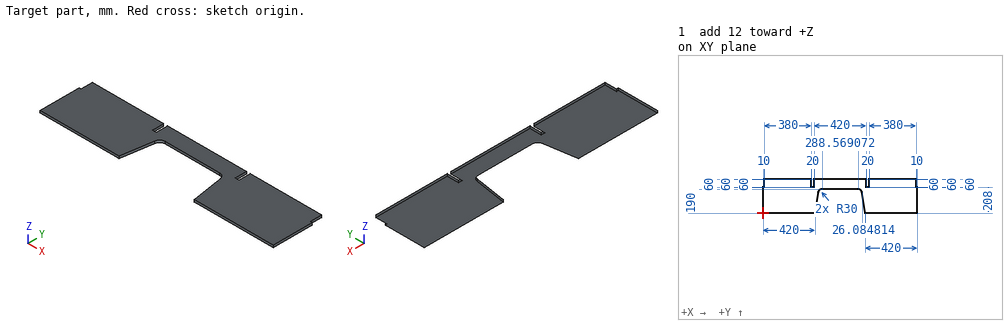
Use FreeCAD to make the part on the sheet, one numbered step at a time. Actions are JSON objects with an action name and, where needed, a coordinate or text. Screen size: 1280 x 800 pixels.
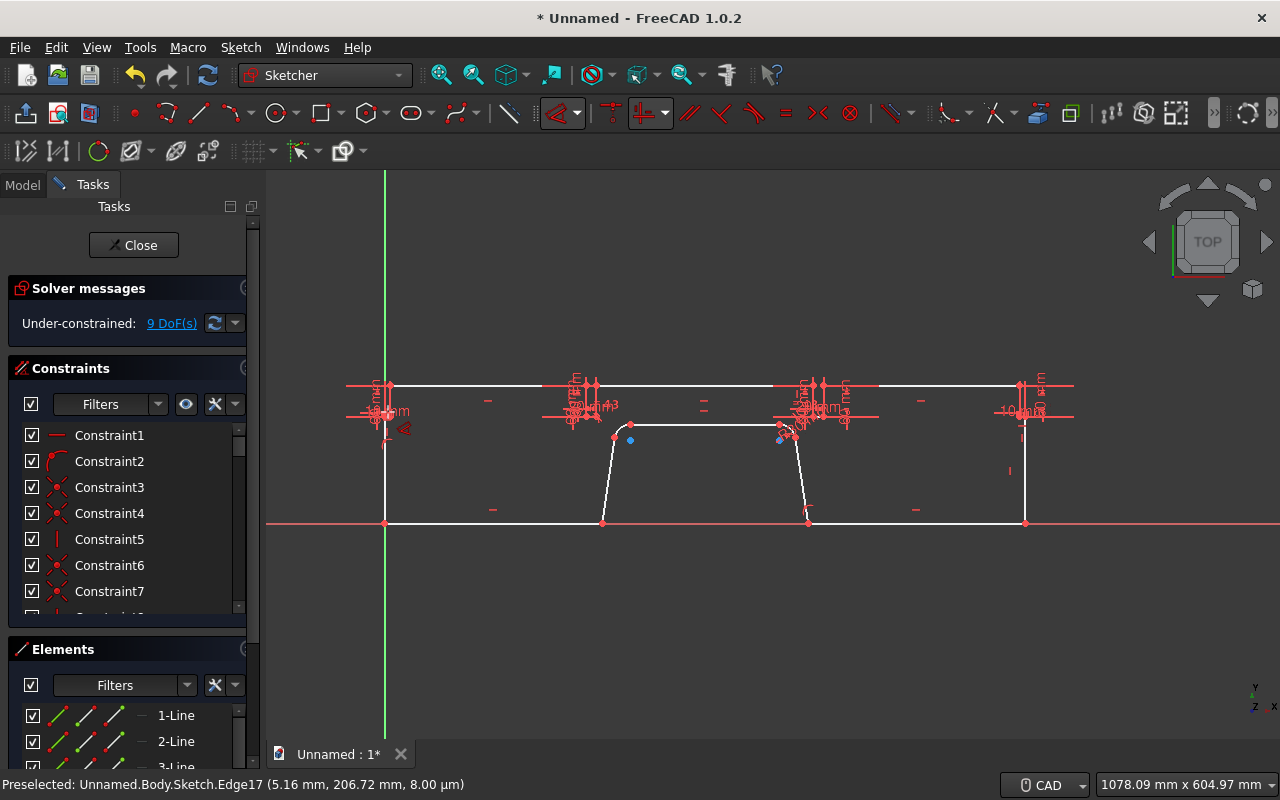
{"action": "left_click", "coordinate": [873, 524]}
{"action": "left_click", "coordinate": [917, 558]}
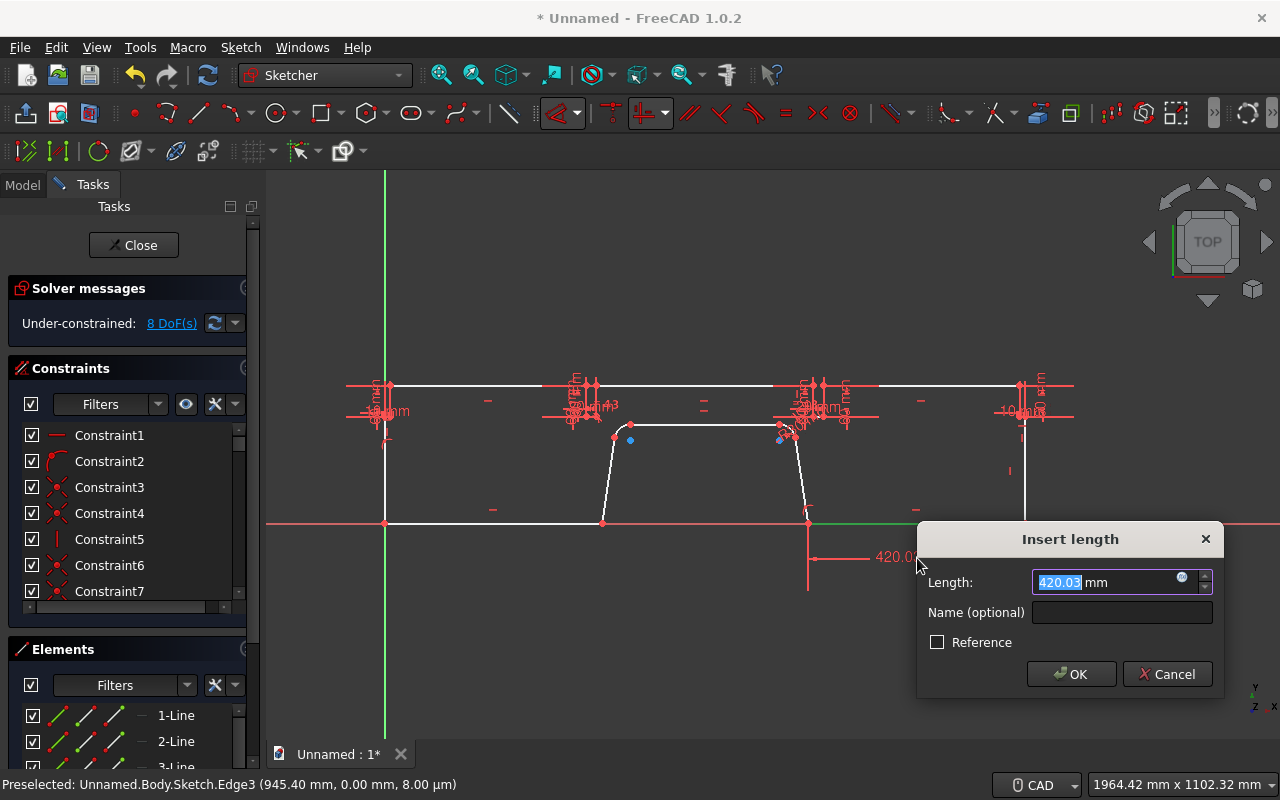
{"action": "type", "text": "420"}
{"action": "key", "text": "Return"}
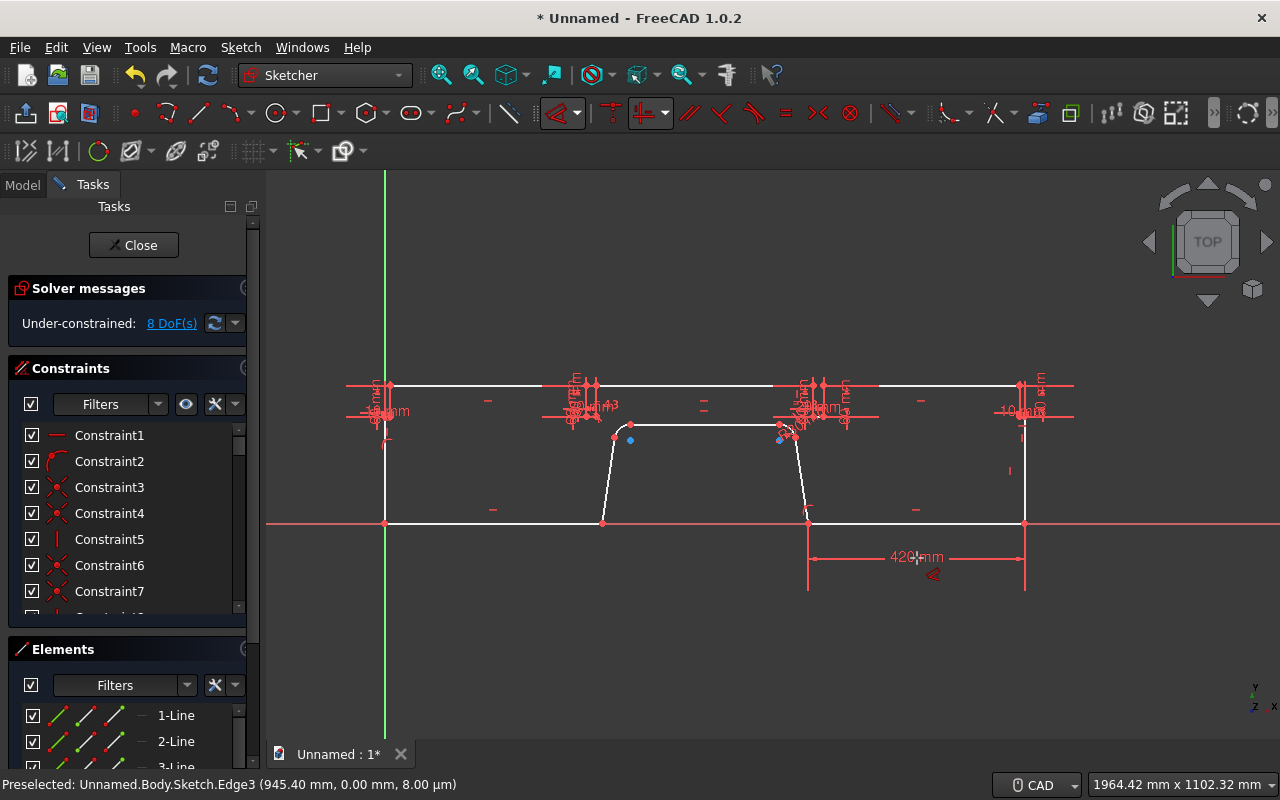
{"action": "left_click", "coordinate": [1025, 492]}
{"action": "left_click", "coordinate": [1059, 470]}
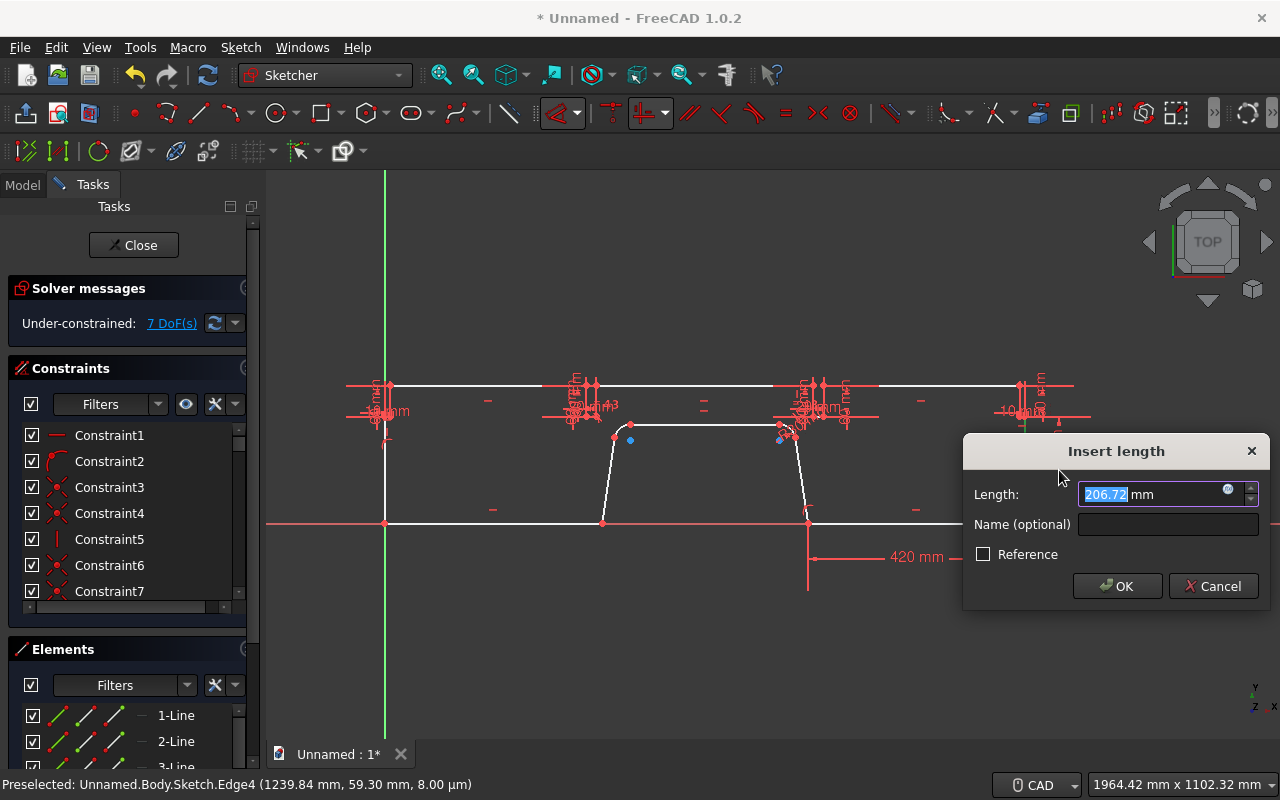
{"action": "type", "text": "208"}
{"action": "key", "text": "Return"}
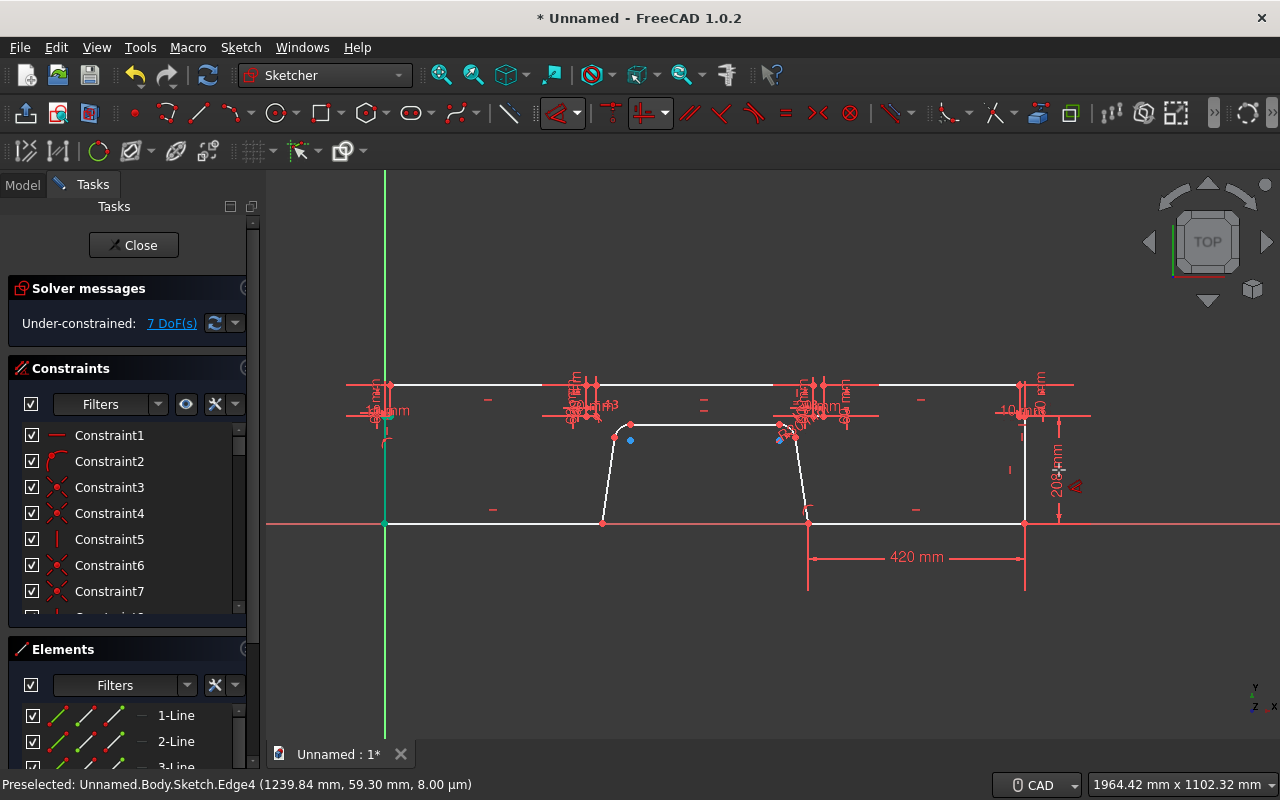
{"action": "left_click", "coordinate": [961, 385]}
{"action": "left_click", "coordinate": [922, 351]}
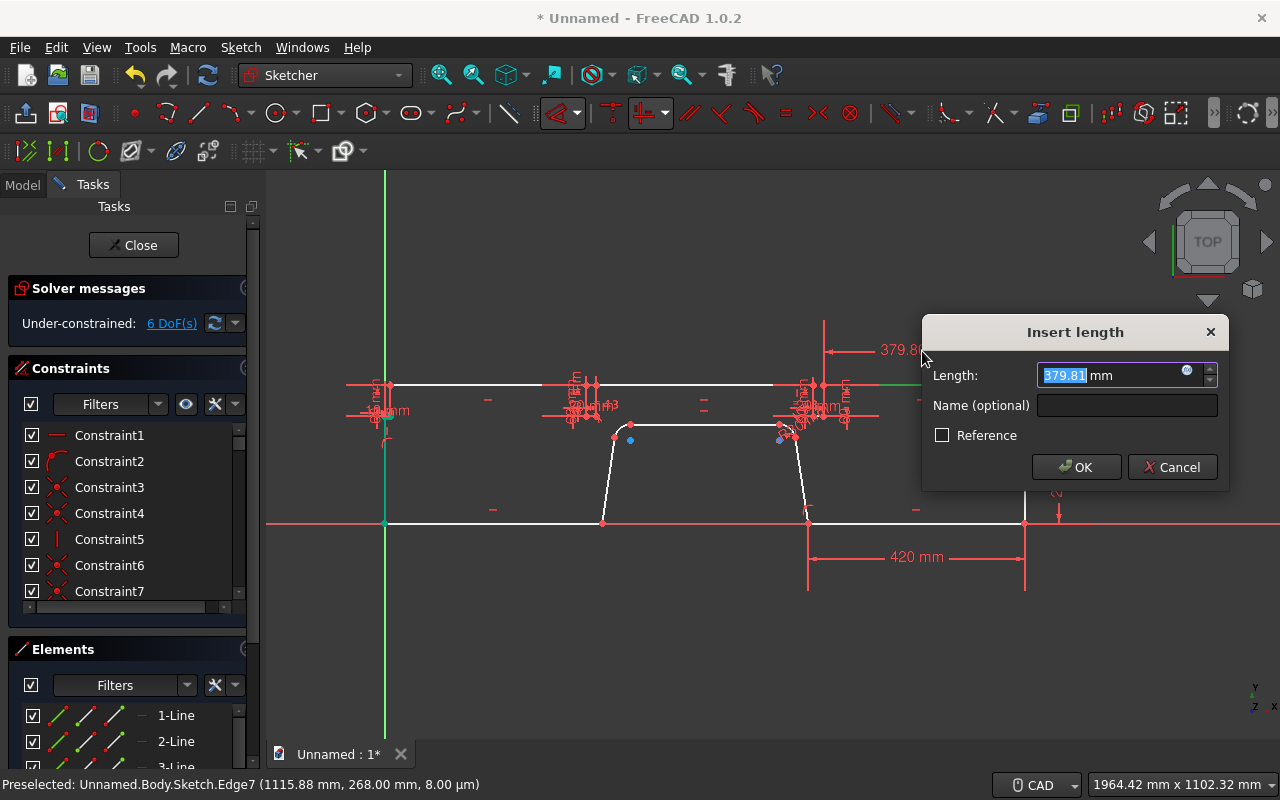
{"action": "type", "text": "380"}
{"action": "key", "text": "Return"}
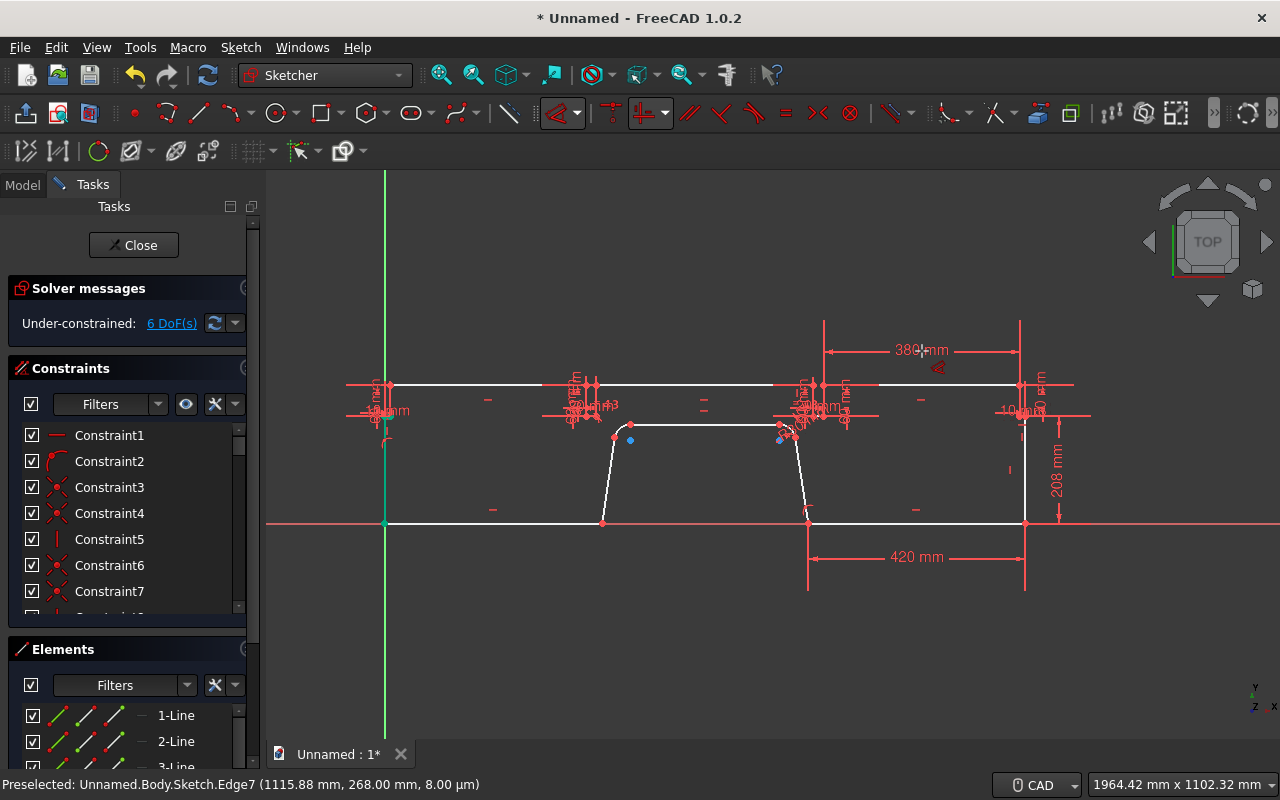
{"action": "left_click", "coordinate": [748, 385]}
{"action": "left_click", "coordinate": [705, 351]}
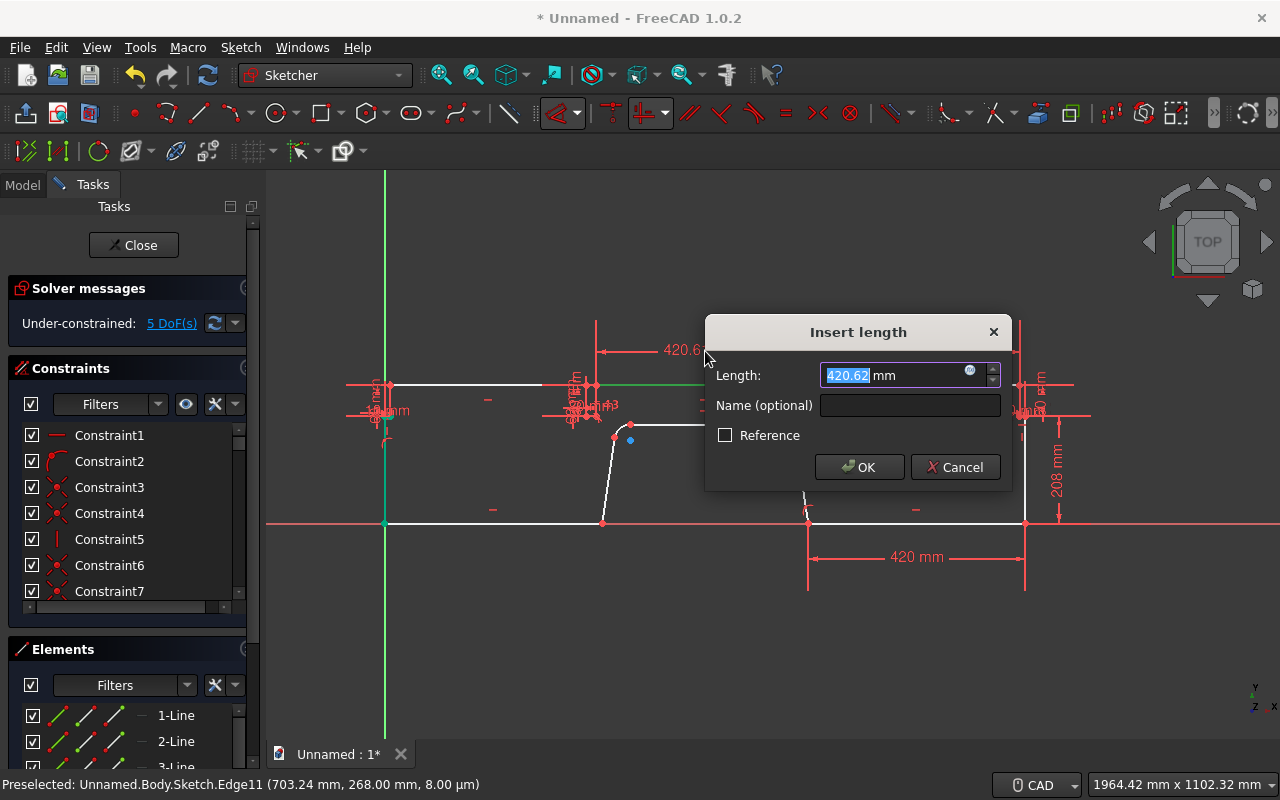
{"action": "type", "text": "420"}
{"action": "key", "text": "Return"}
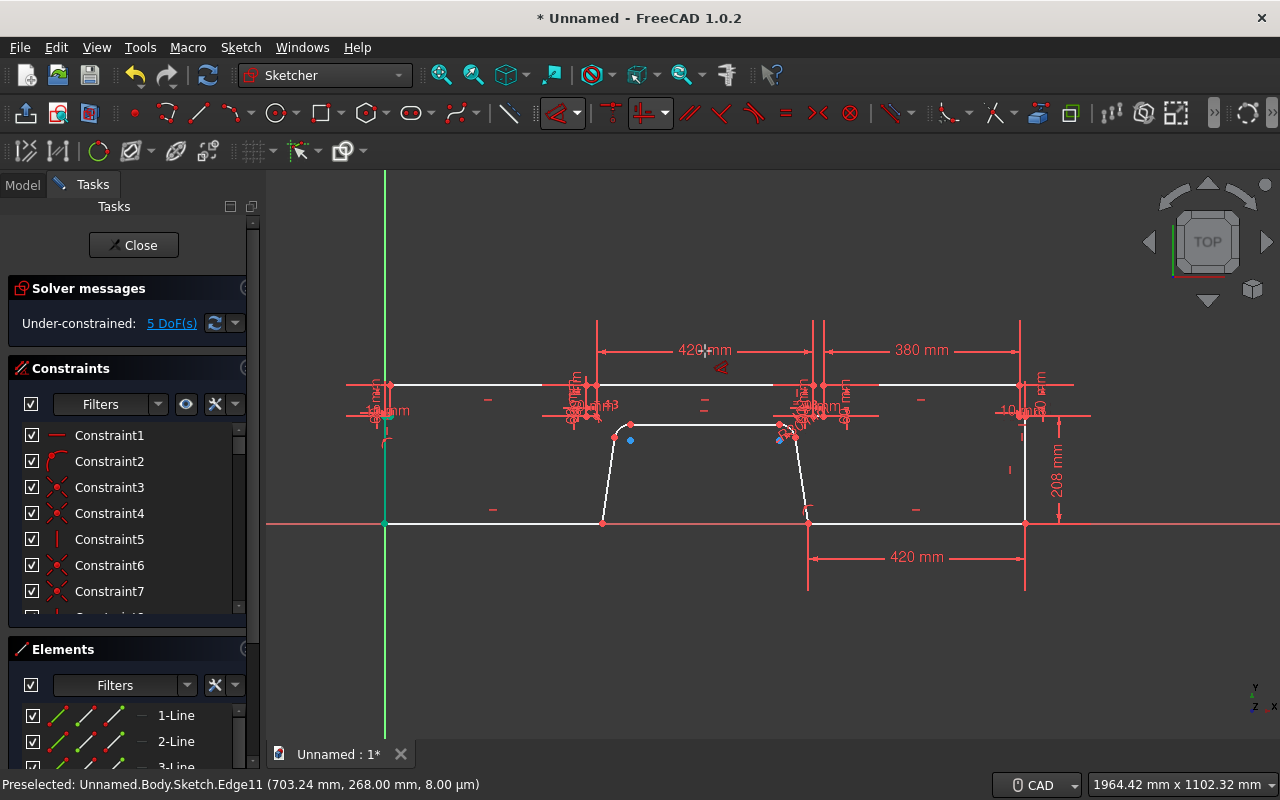
{"action": "left_click", "coordinate": [527, 385]}
{"action": "left_click", "coordinate": [488, 351]}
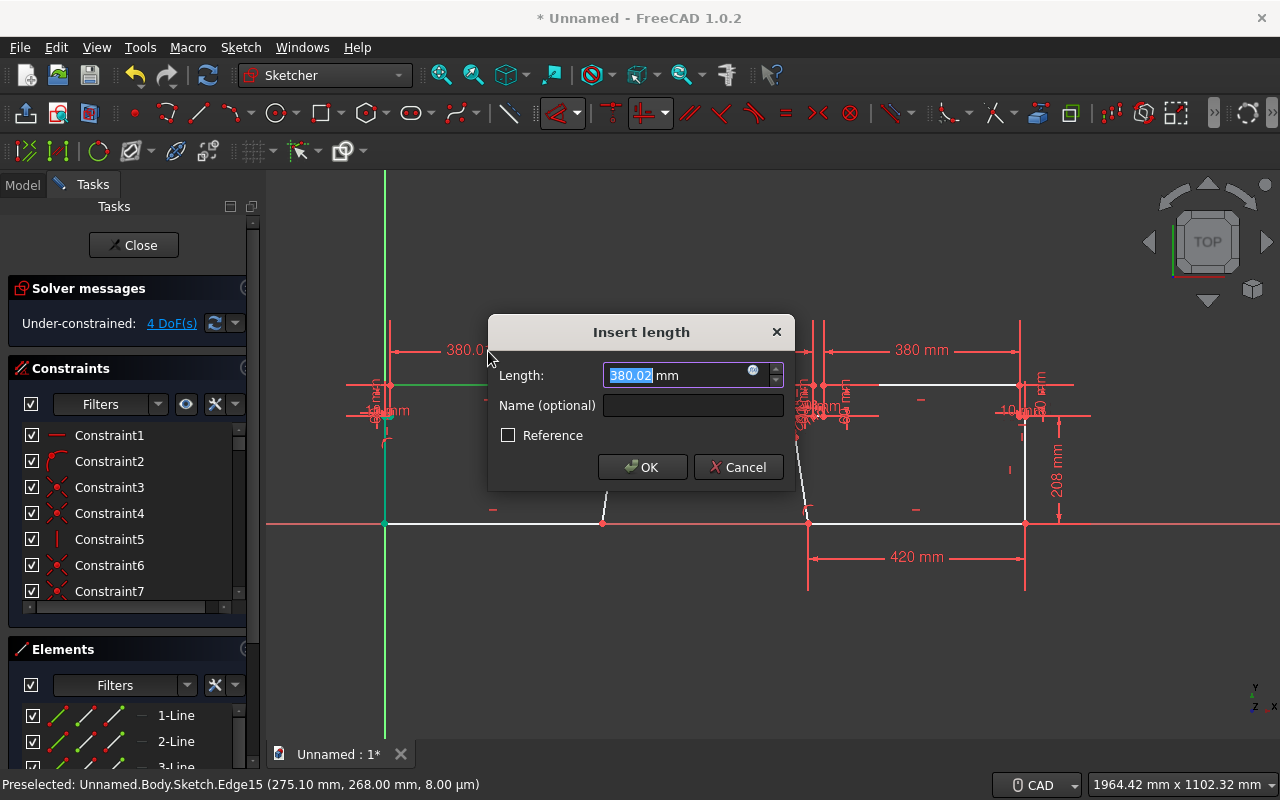
{"action": "type", "text": "380"}
{"action": "key", "text": "Return"}